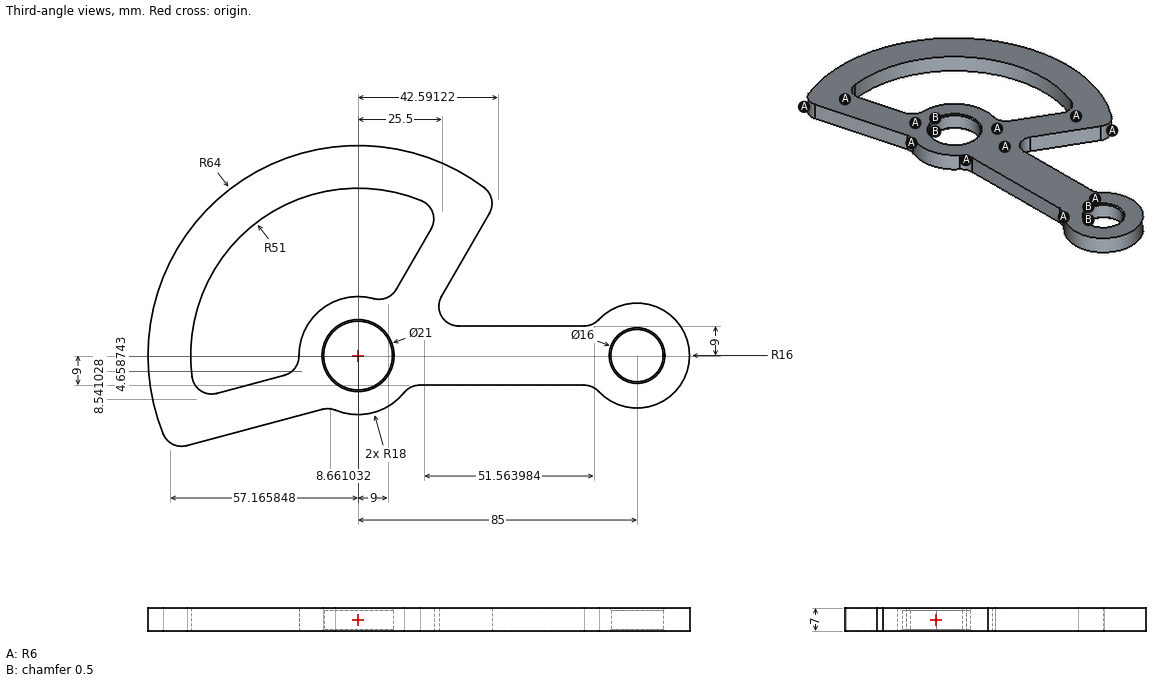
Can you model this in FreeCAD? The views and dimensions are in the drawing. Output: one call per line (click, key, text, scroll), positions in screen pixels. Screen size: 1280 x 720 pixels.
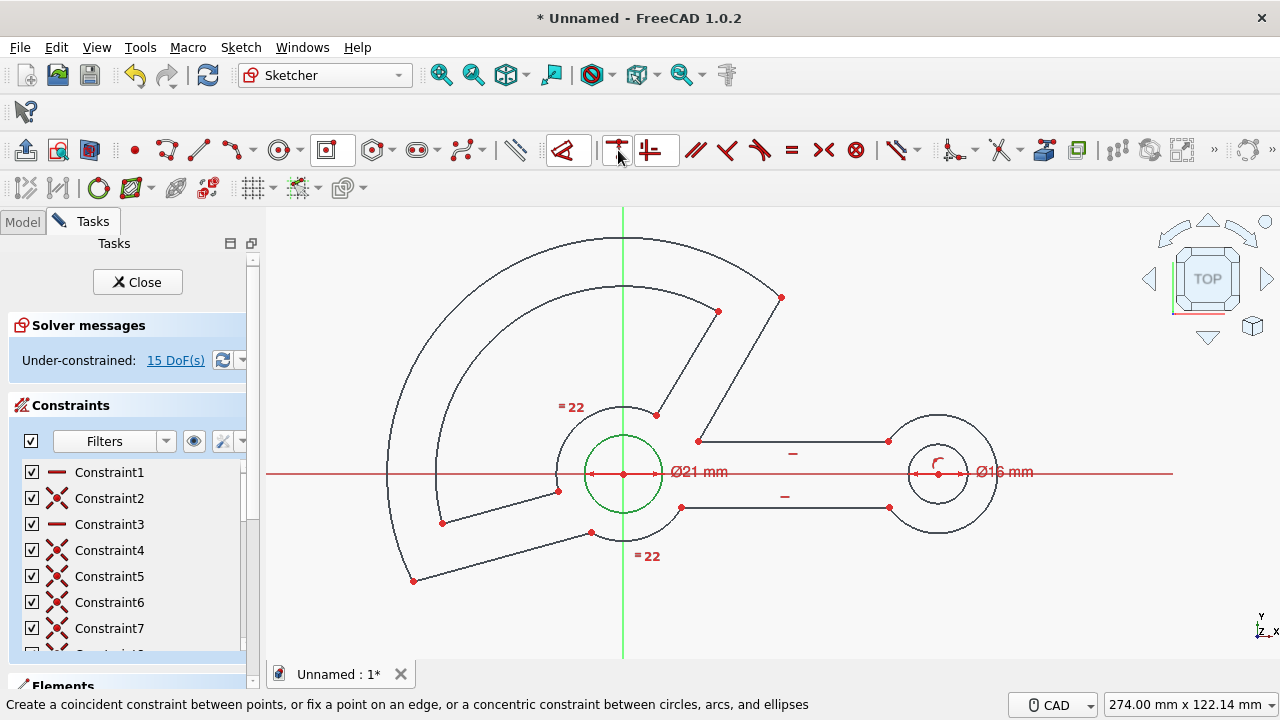
click(562, 150)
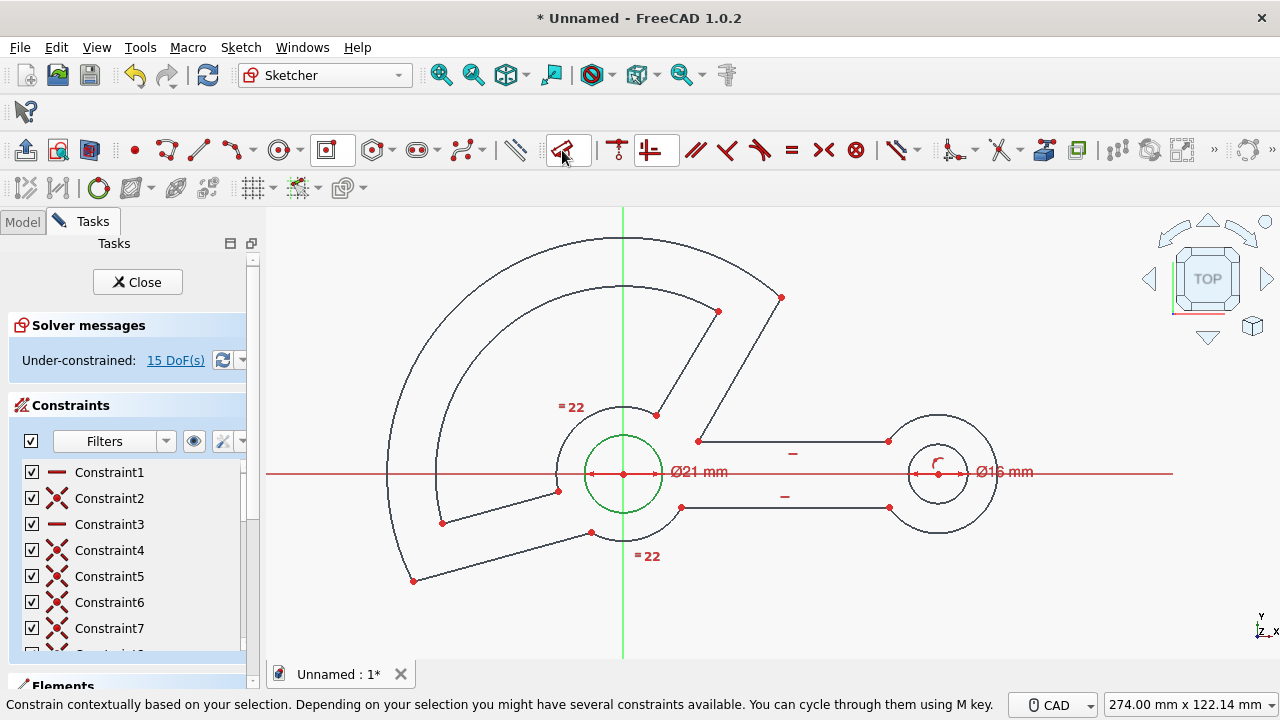
click(599, 239)
click(471, 253)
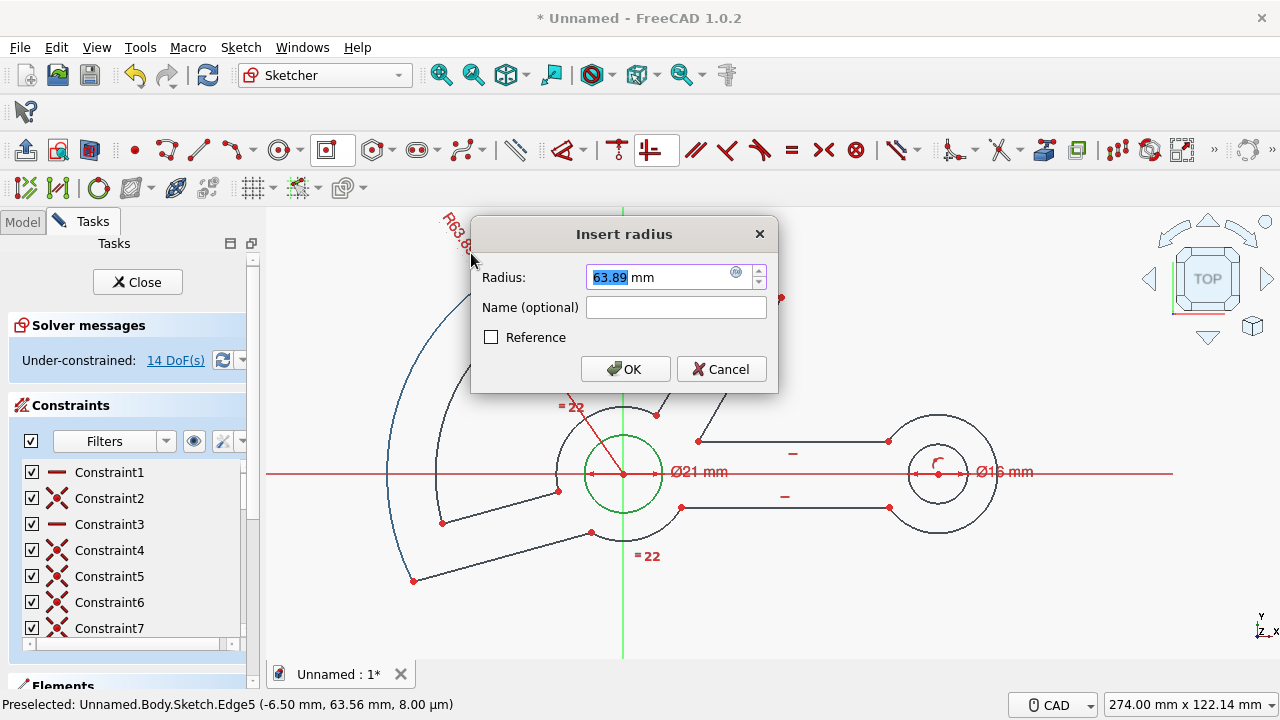
text(64)
key(Return)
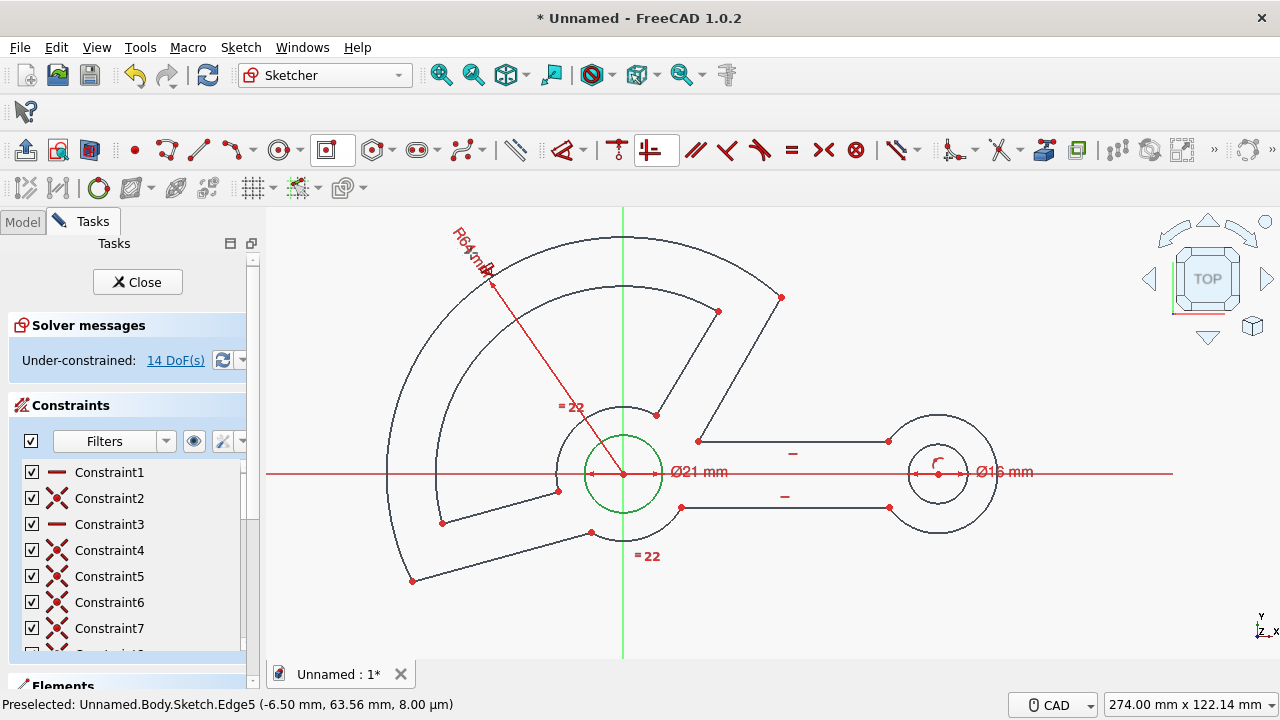
click(621, 541)
click(573, 559)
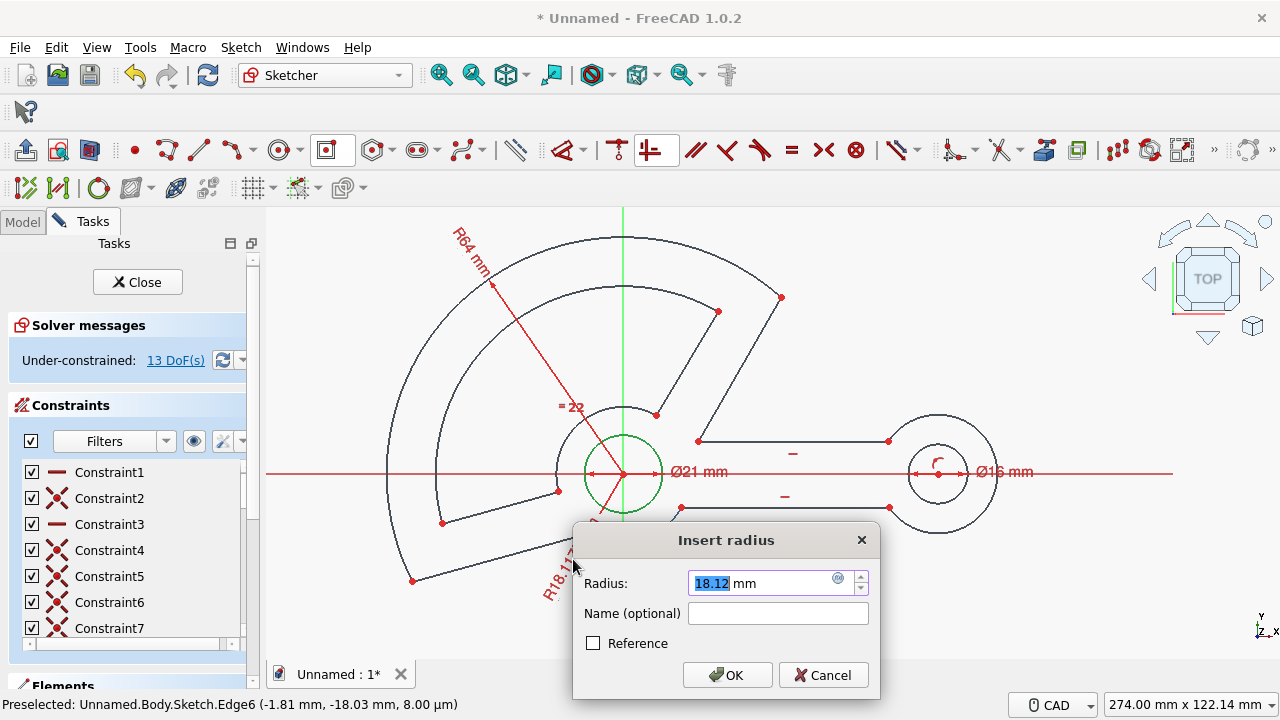
text(18)
key(Return)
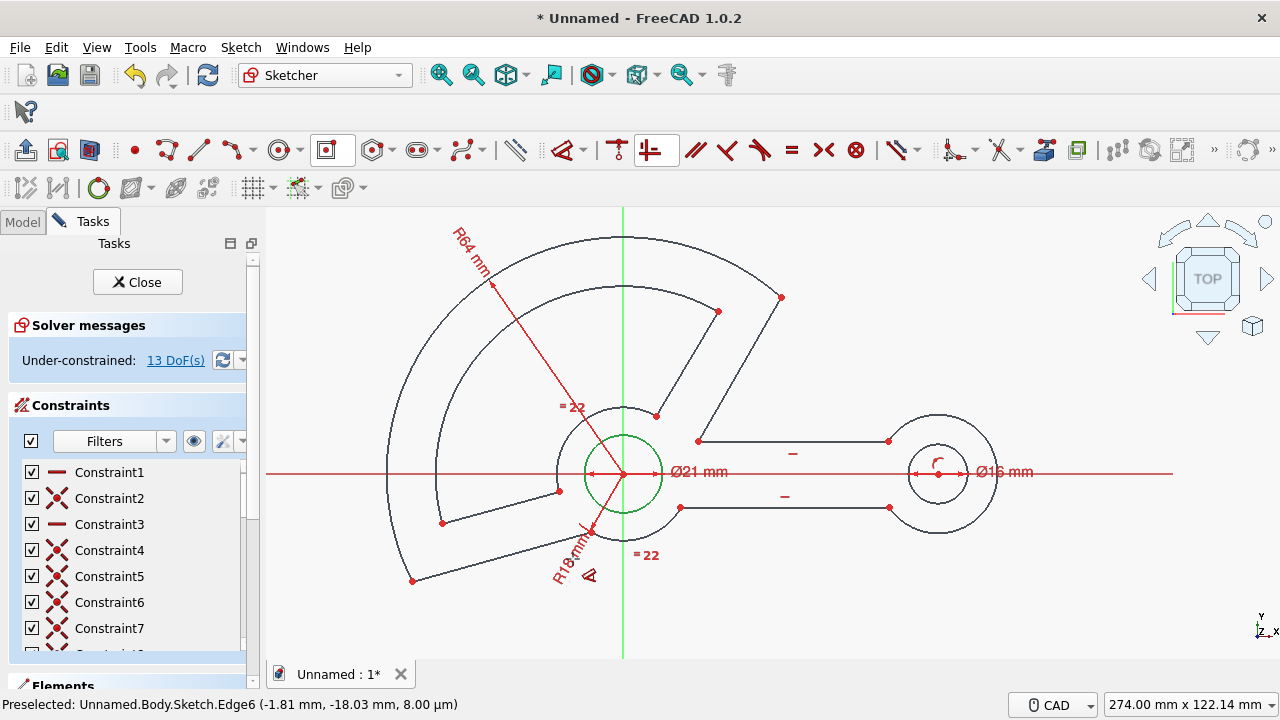
click(970, 524)
click(987, 551)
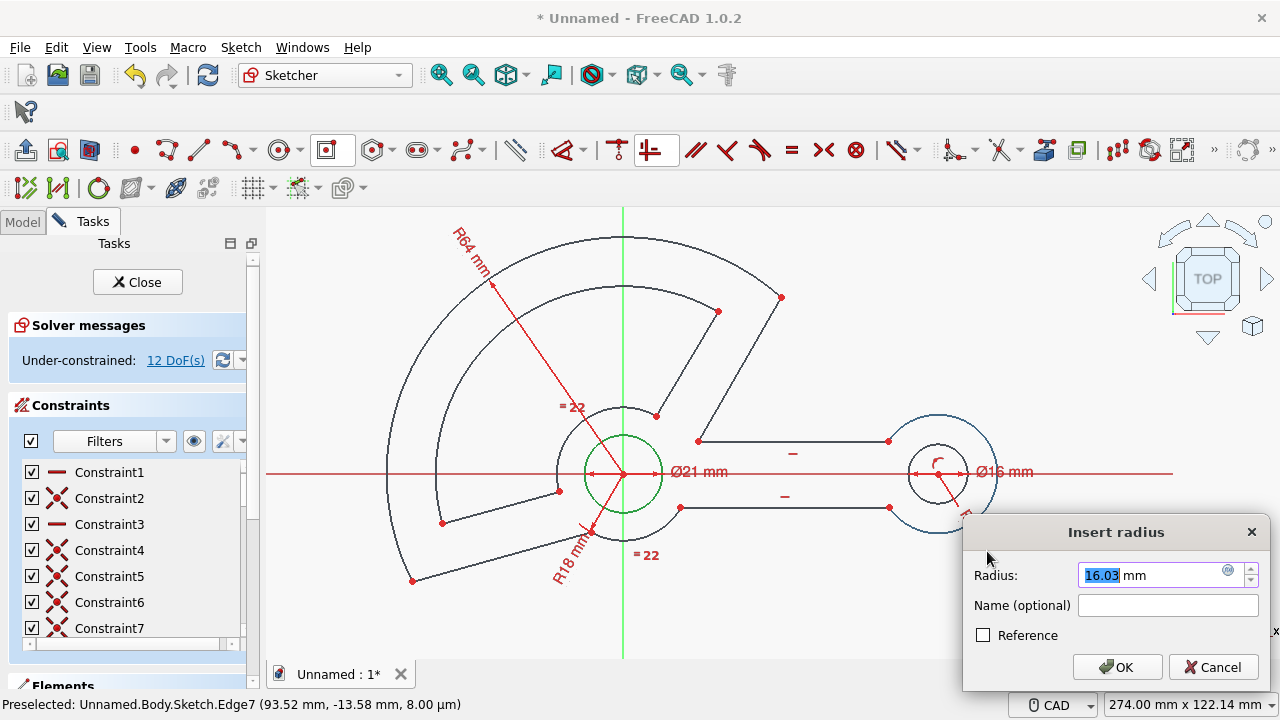
text(16)
key(Return)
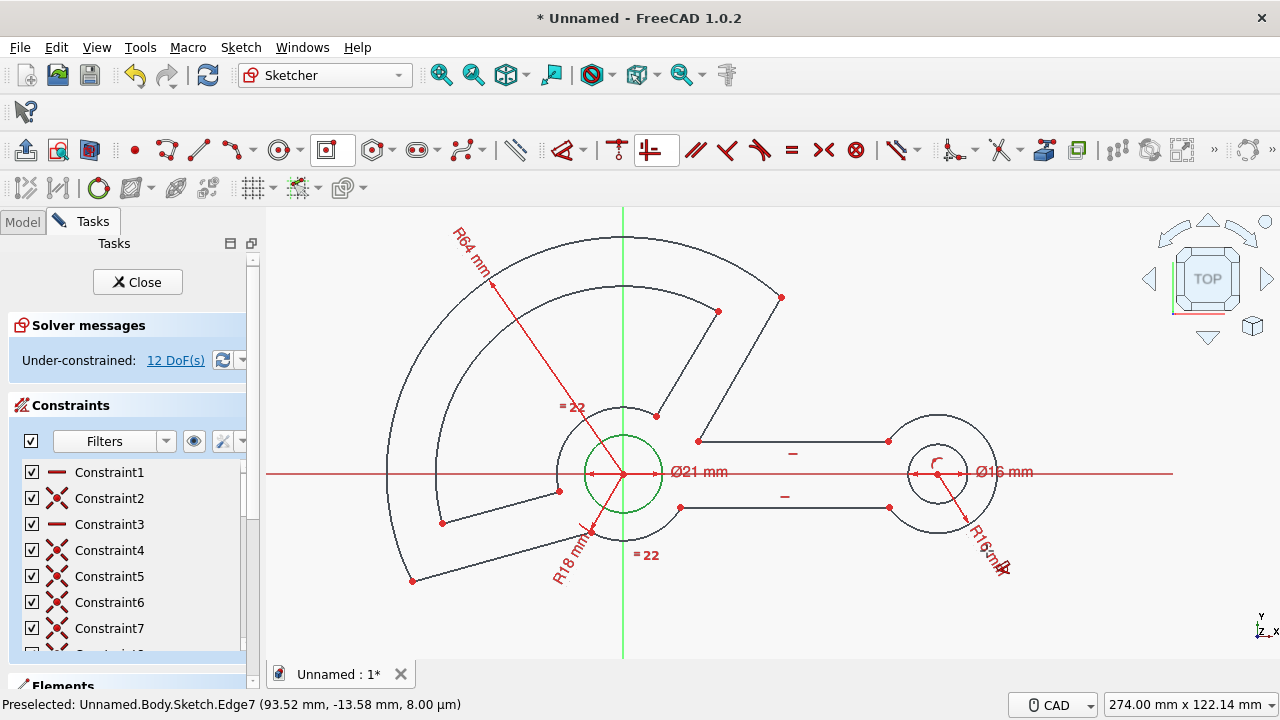
click(590, 289)
click(584, 258)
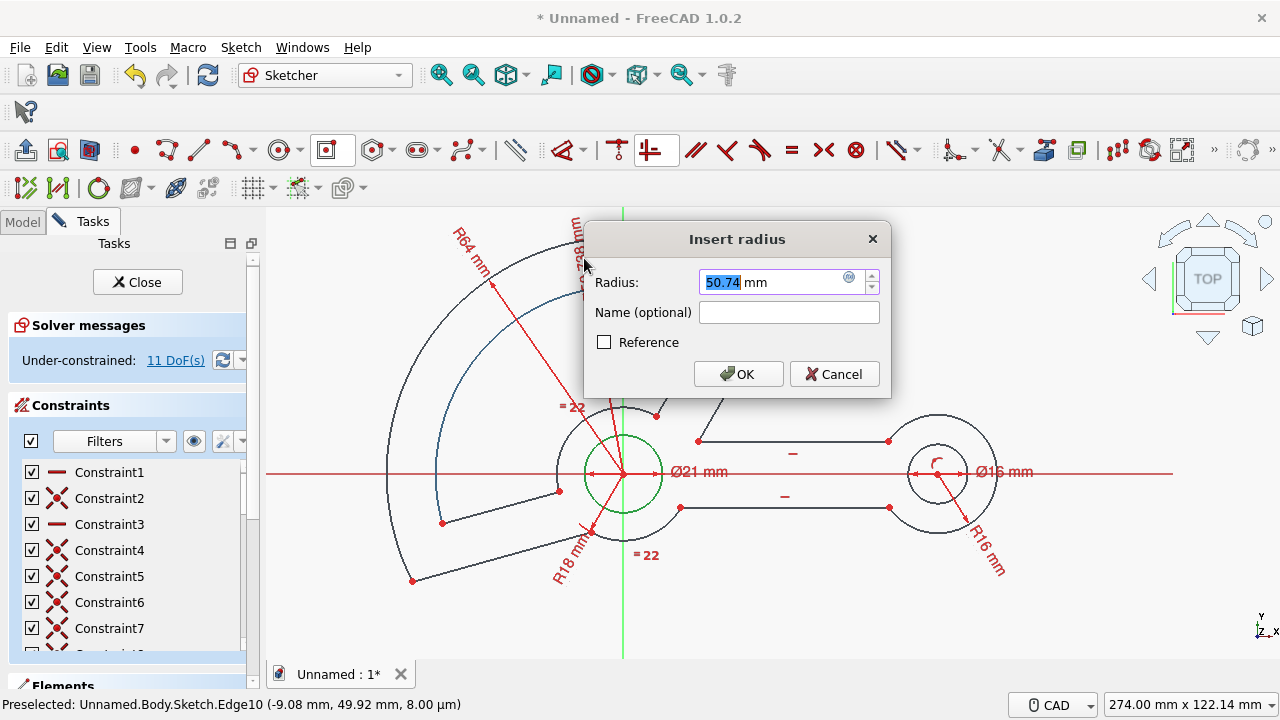
text(51)
key(Return)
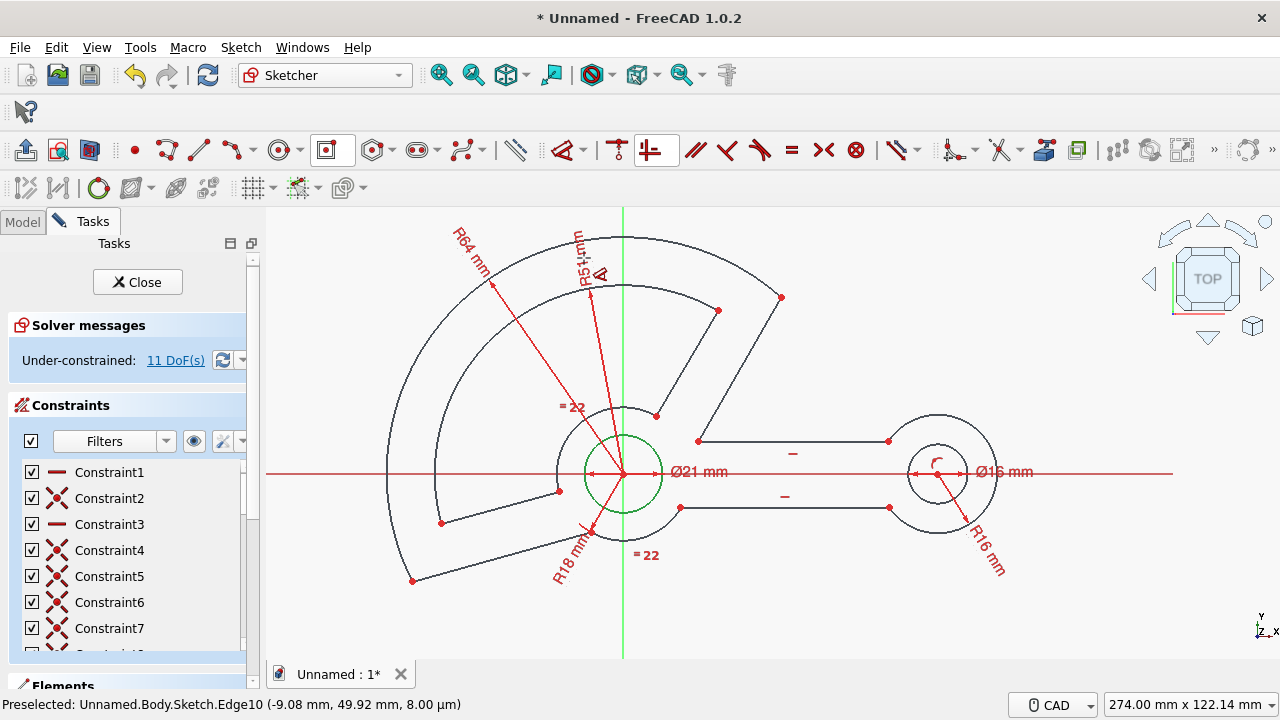
click(888, 442)
click(541, 458)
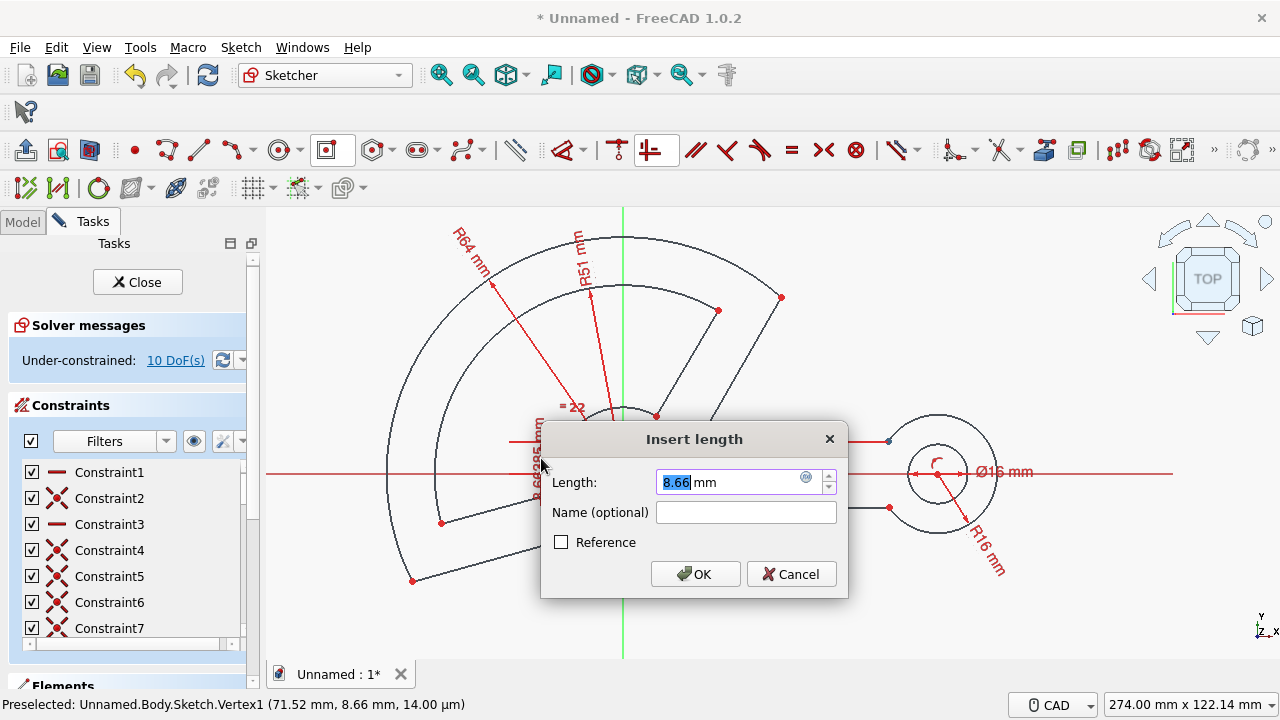
text(9)
key(Return)